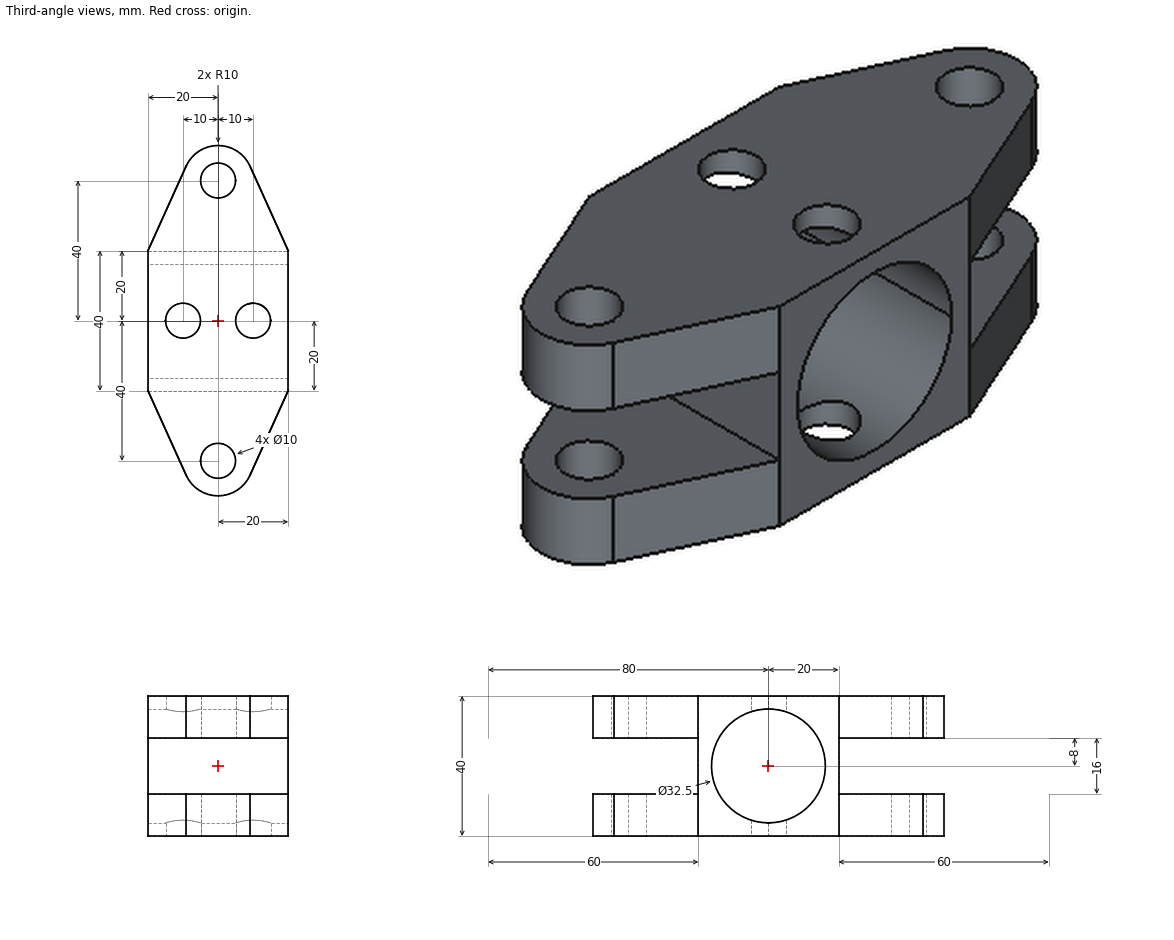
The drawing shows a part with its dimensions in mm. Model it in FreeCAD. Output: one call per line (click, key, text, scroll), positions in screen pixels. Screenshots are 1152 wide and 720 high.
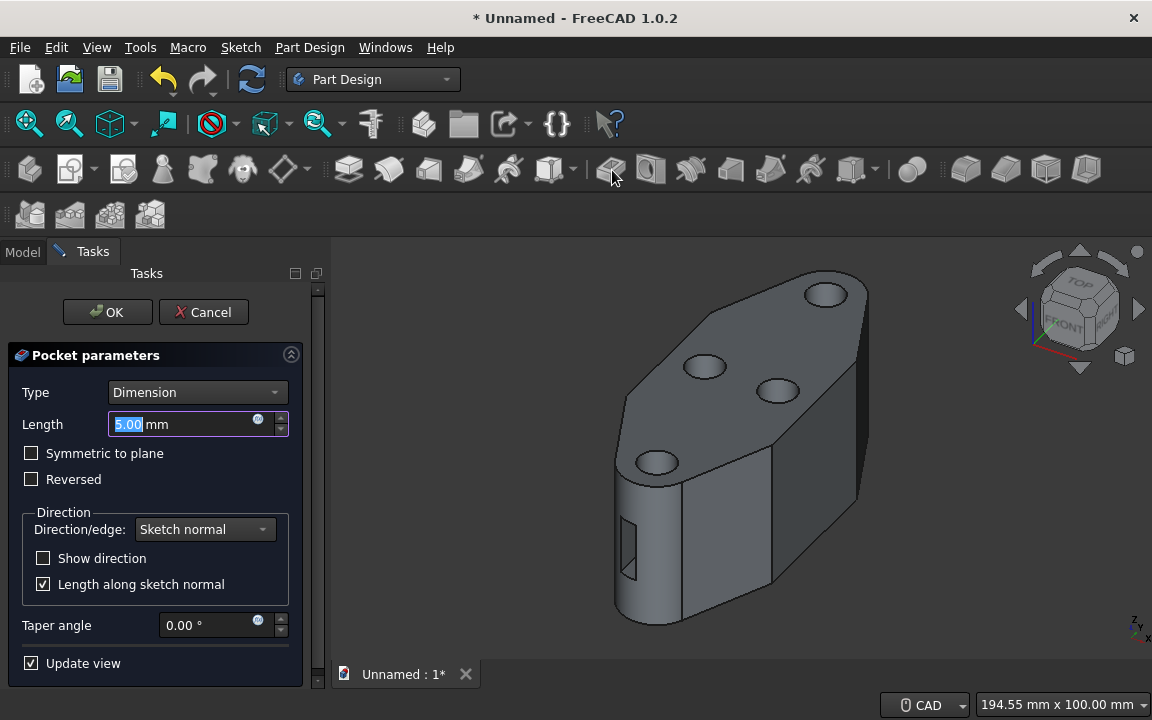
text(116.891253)
key(Tab)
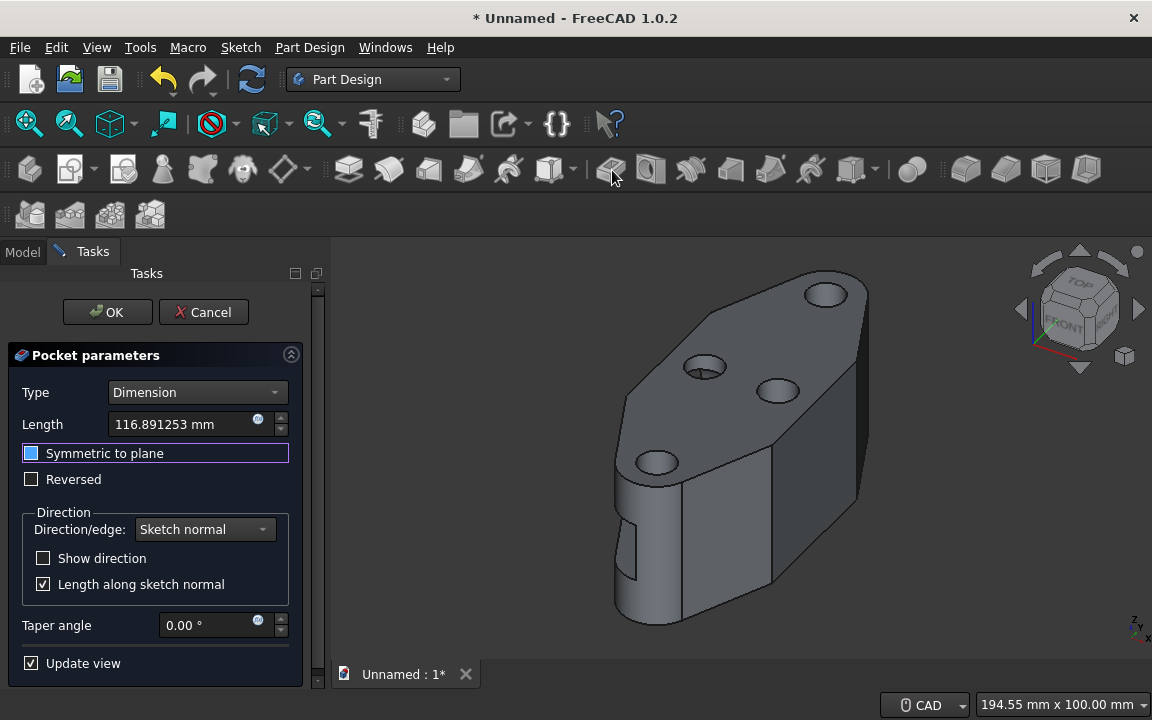
click(30, 453)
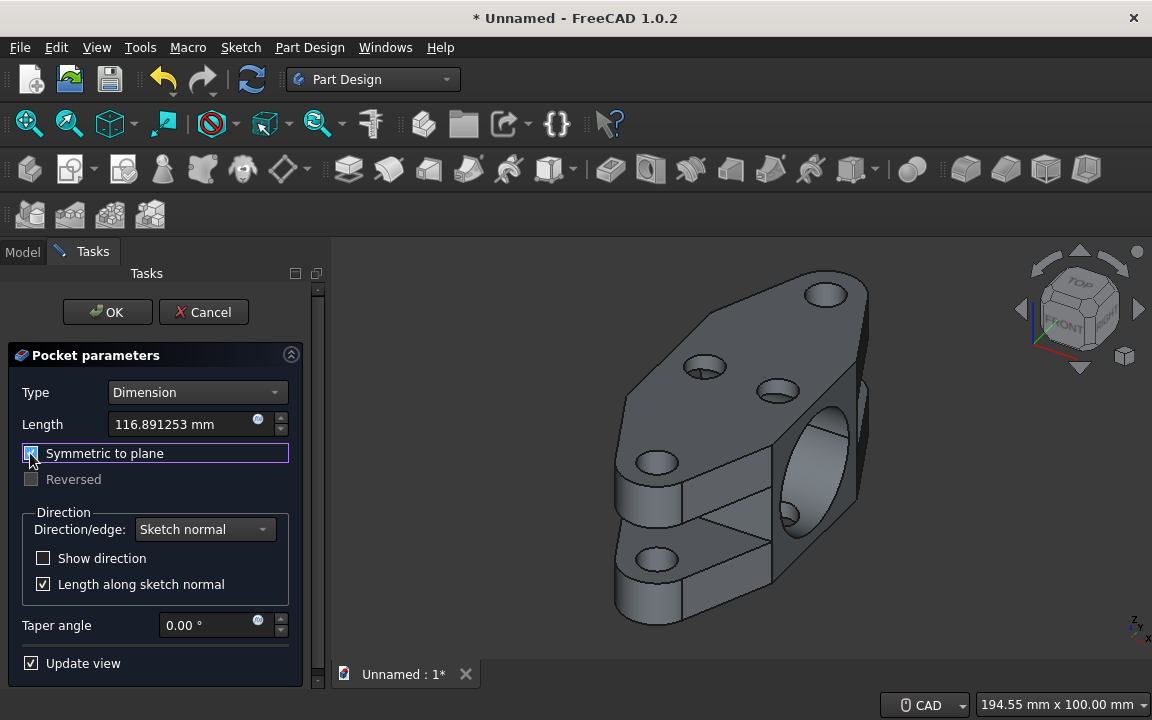
click(108, 312)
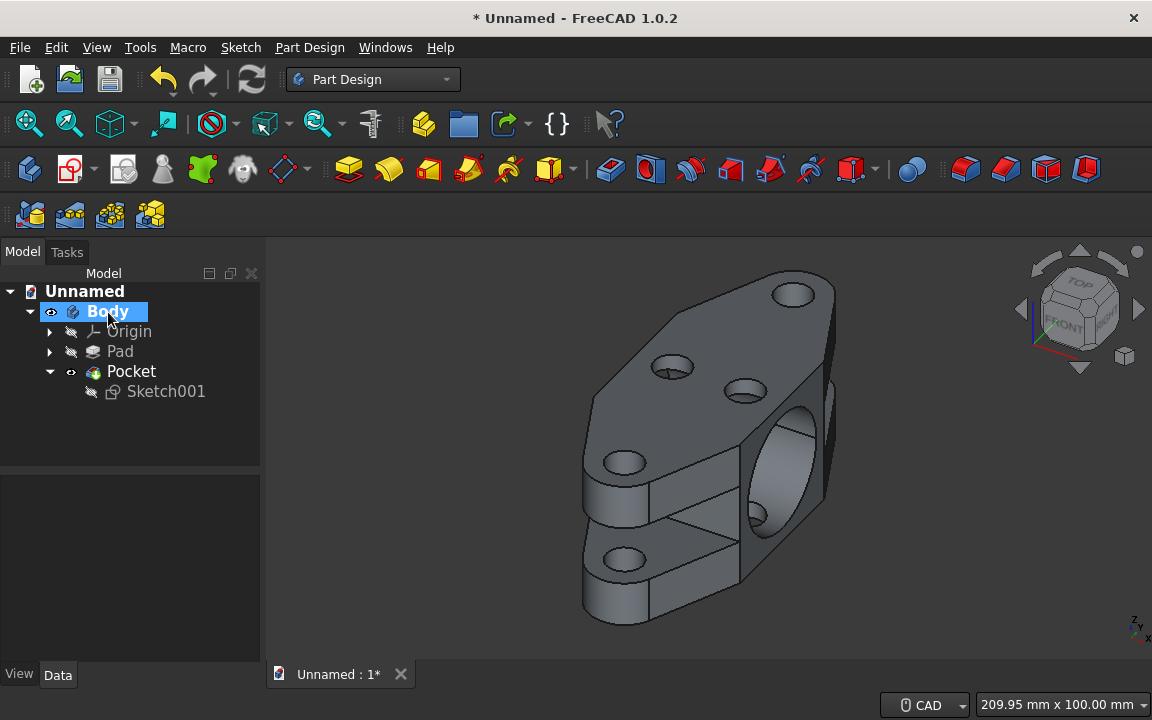
key(0)